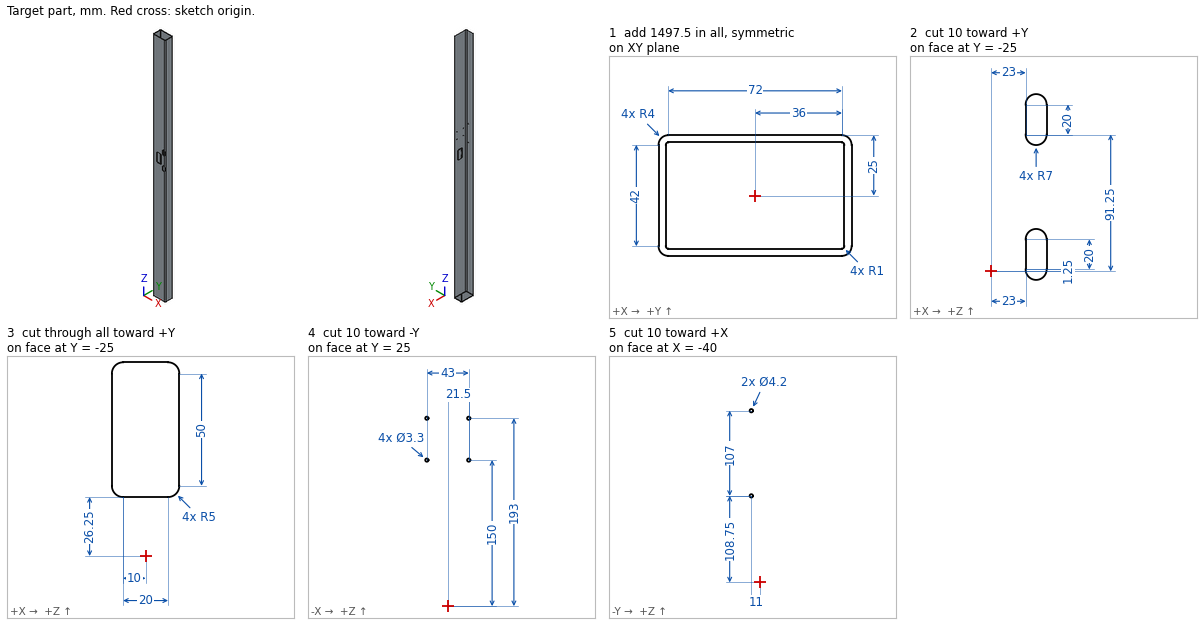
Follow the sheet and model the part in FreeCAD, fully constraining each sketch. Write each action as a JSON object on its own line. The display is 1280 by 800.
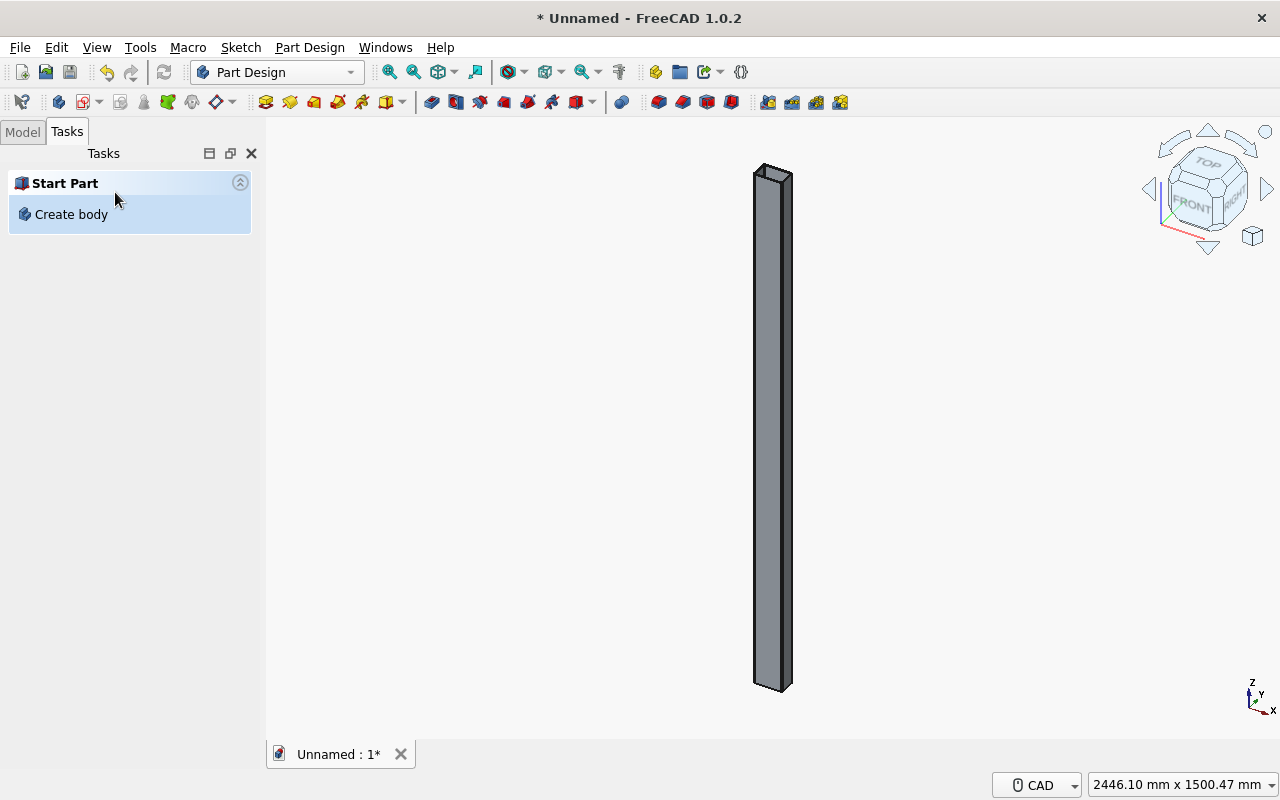
{"action": "left_click", "coordinate": [768, 214]}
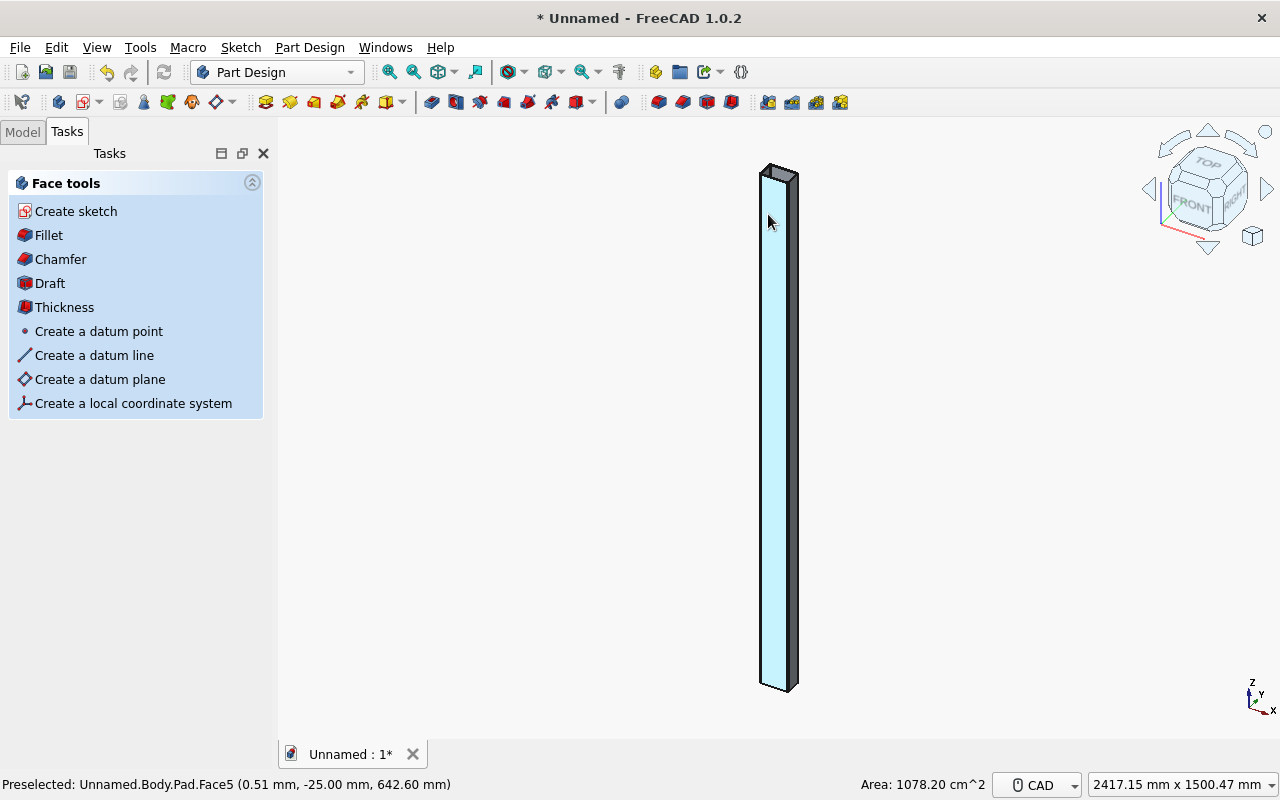
{"action": "left_click", "coordinate": [84, 102]}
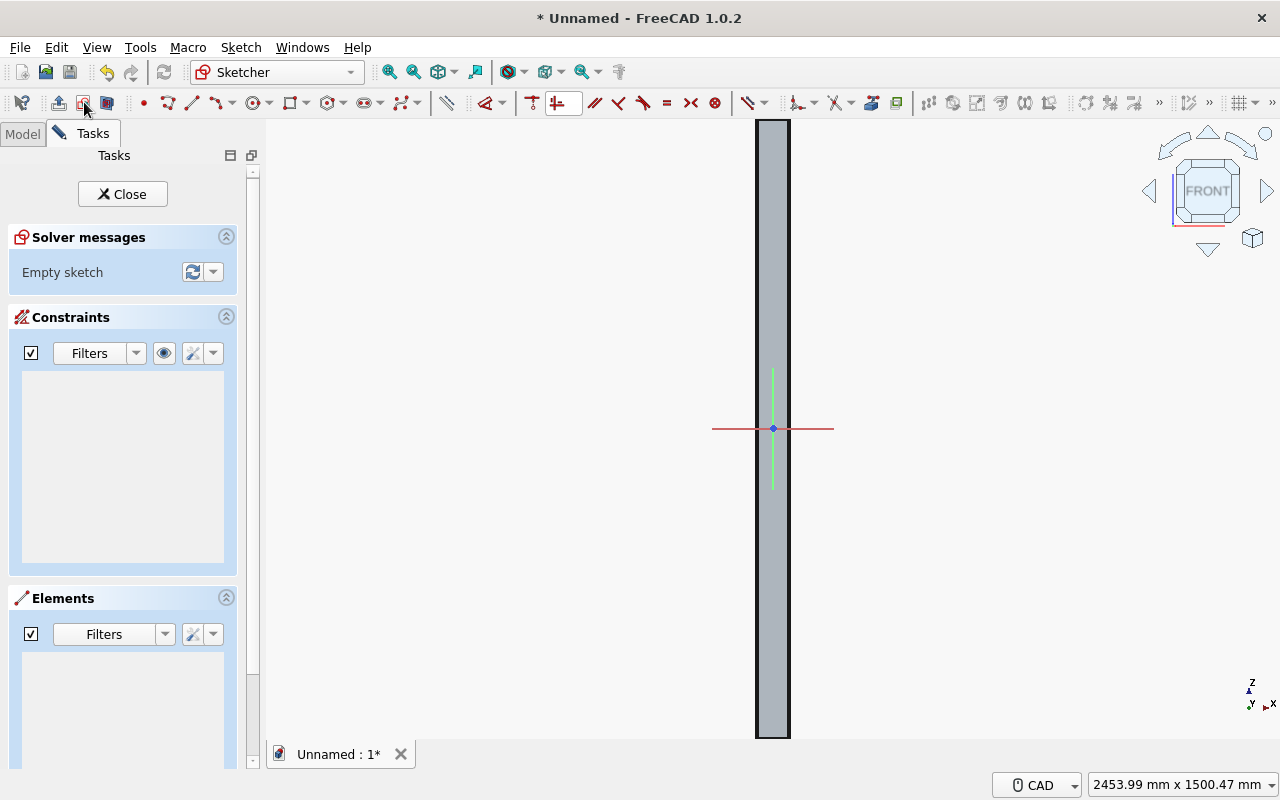
{"action": "scroll", "coordinate": [793, 402], "scroll_direction": "up", "scroll_amount": 10}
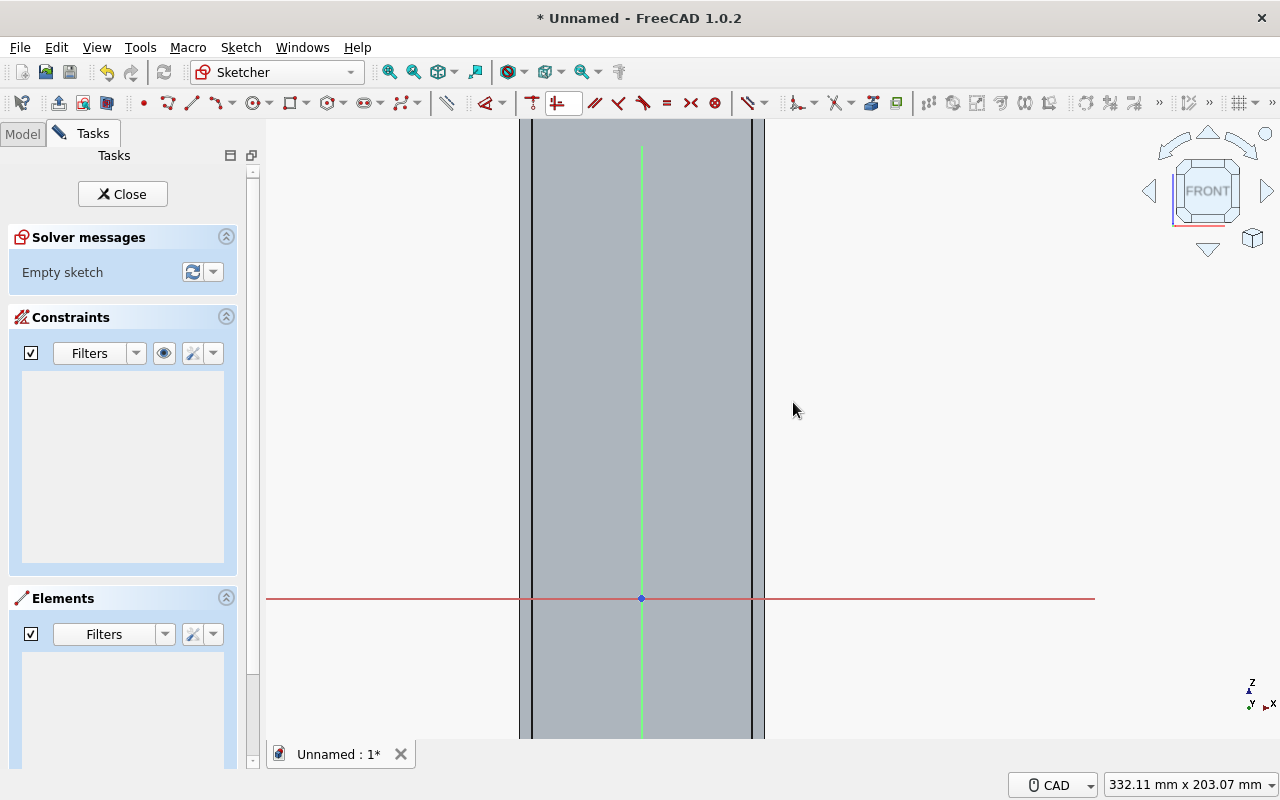
{"action": "key", "text": "g s"}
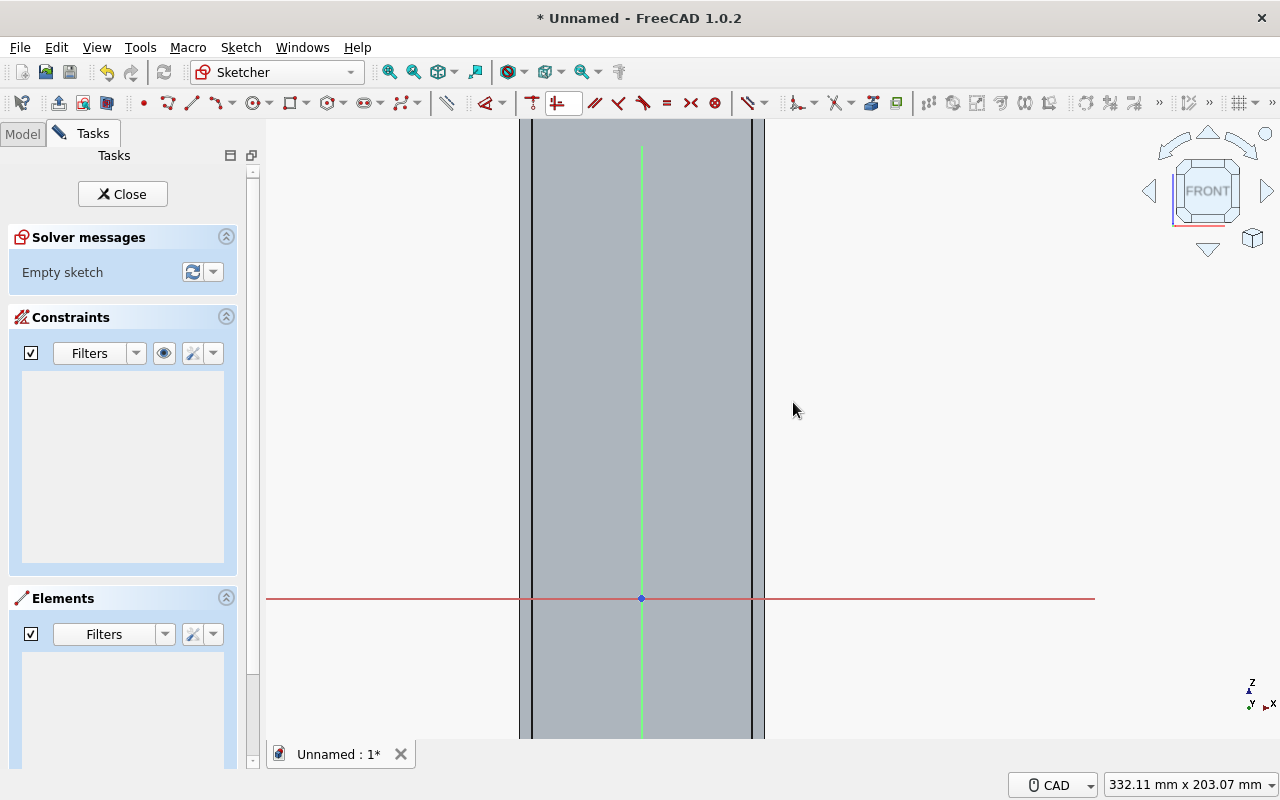
{"action": "left_click", "coordinate": [733, 320]}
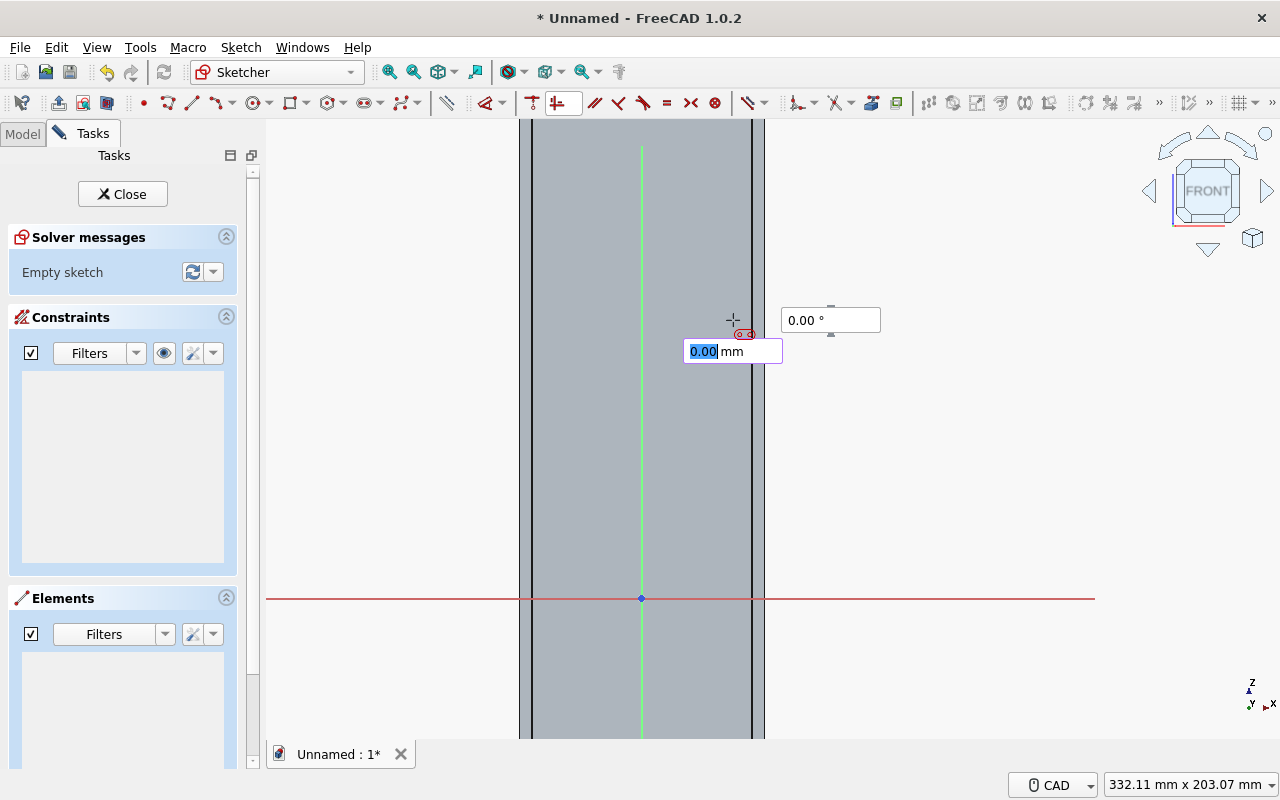
{"action": "left_click", "coordinate": [733, 259]}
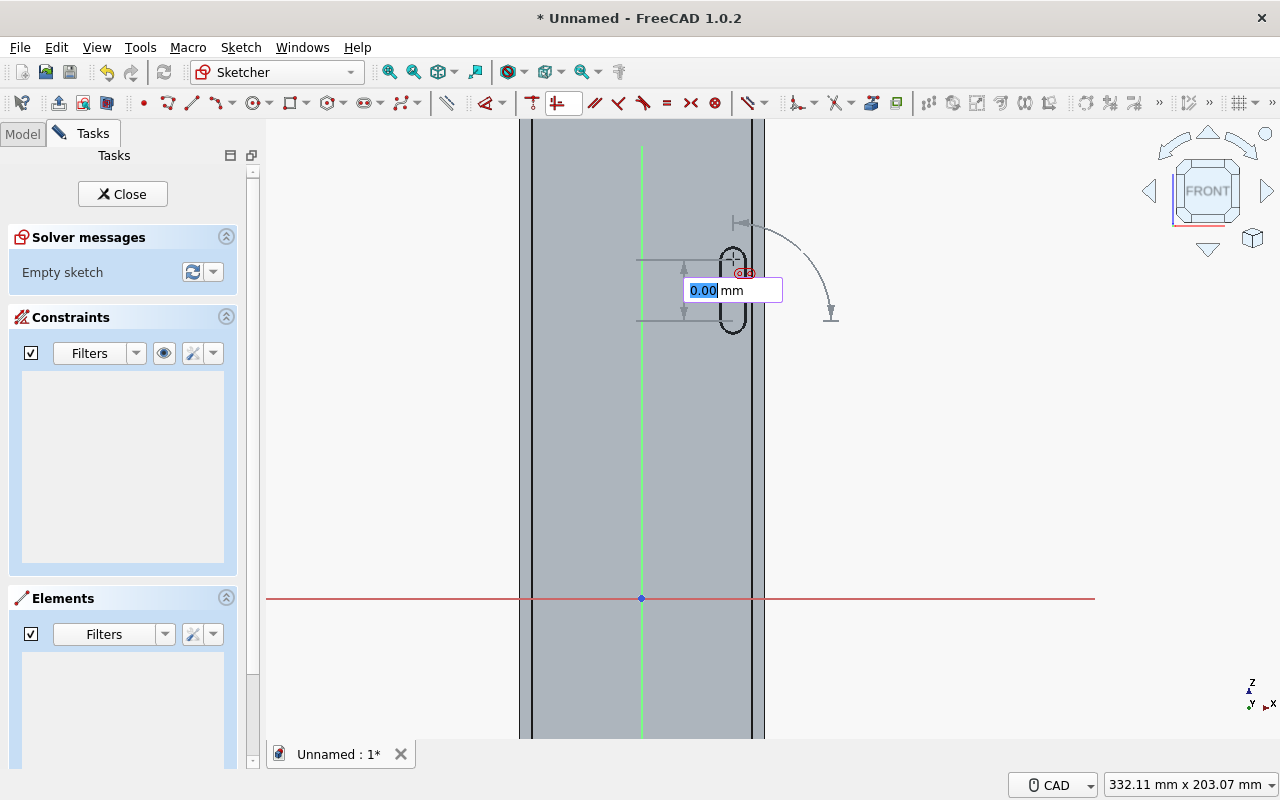
{"action": "left_click", "coordinate": [712, 289]}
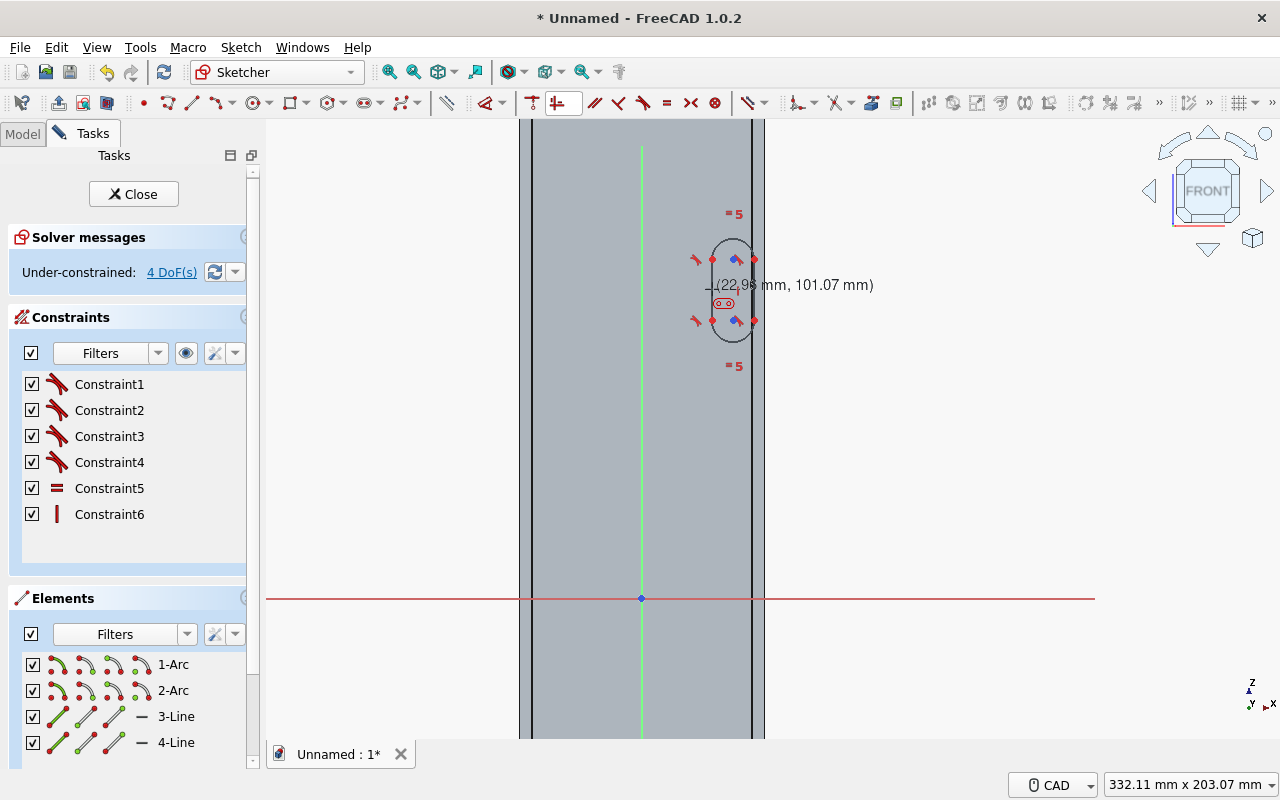
{"action": "scroll", "coordinate": [733, 595], "scroll_direction": "up", "scroll_amount": 8}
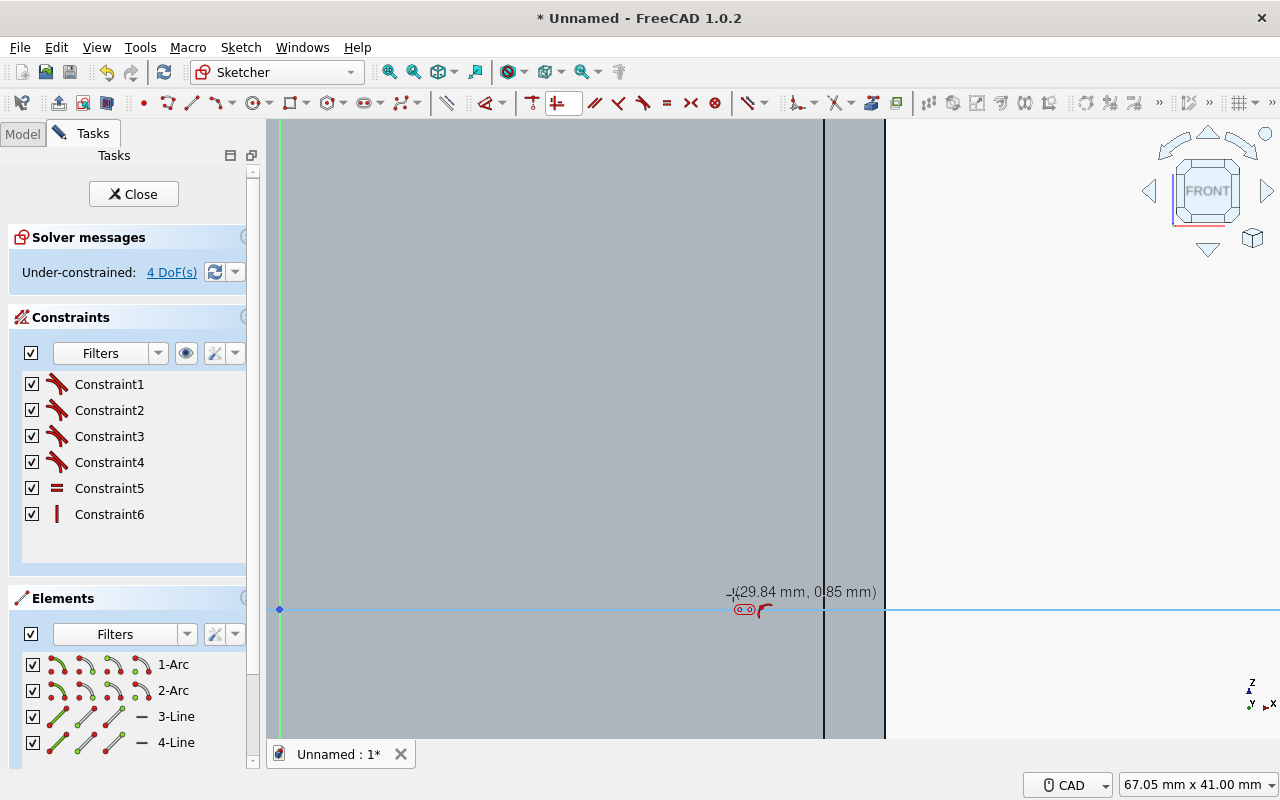
{"action": "left_click", "coordinate": [734, 591]}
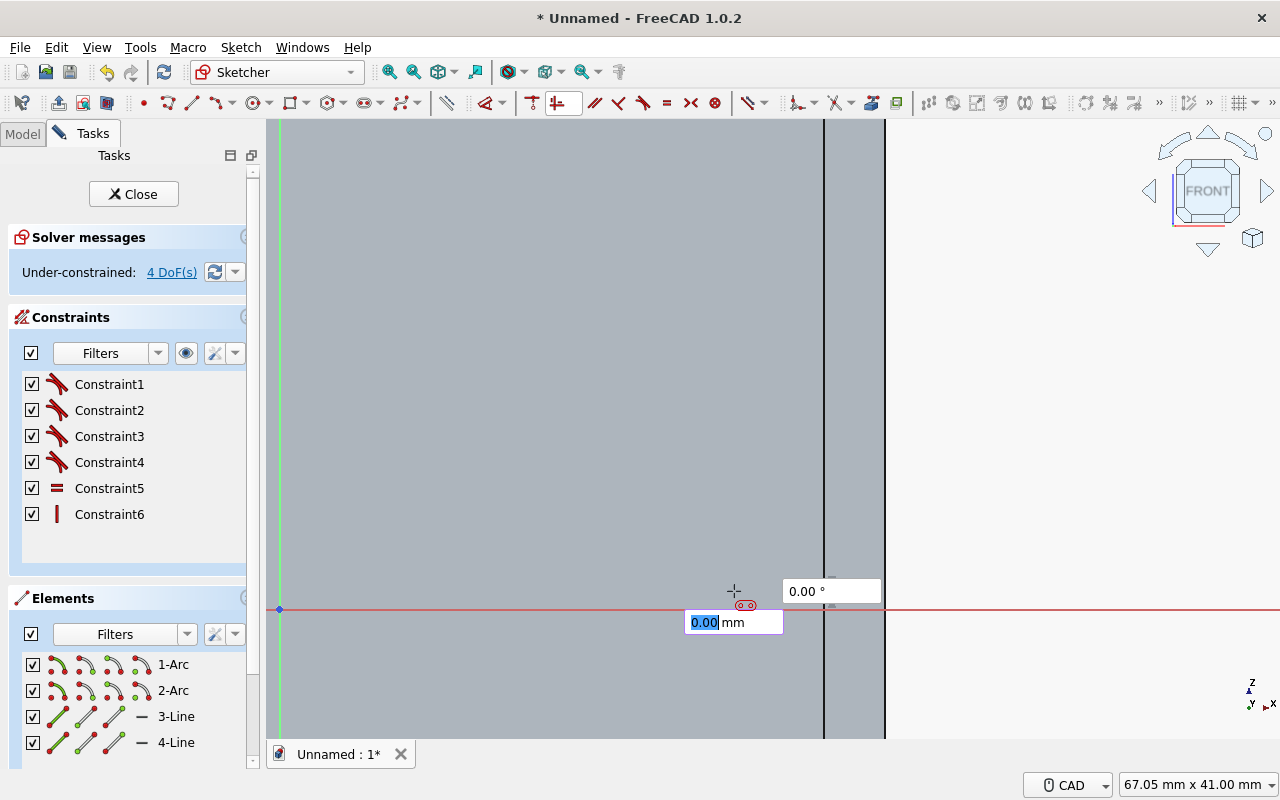
{"action": "scroll", "coordinate": [741, 598], "scroll_direction": "down", "scroll_amount": 8}